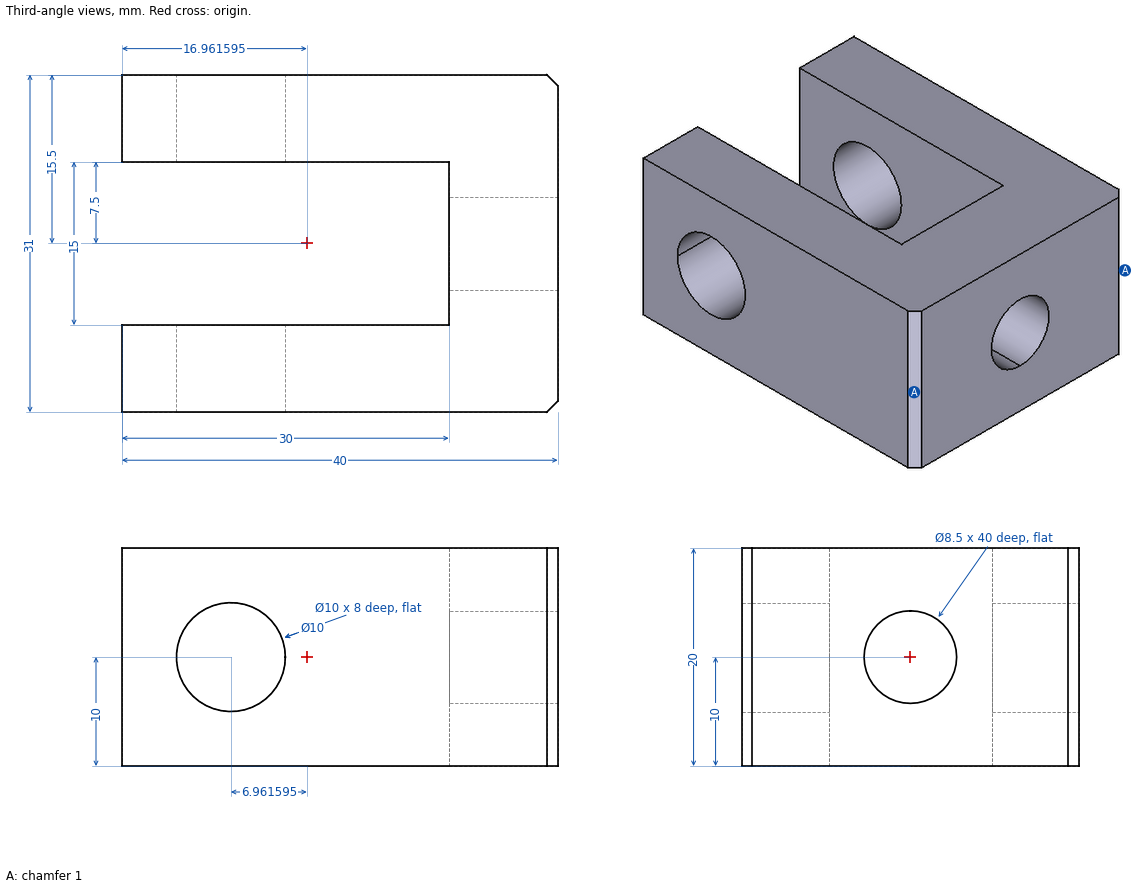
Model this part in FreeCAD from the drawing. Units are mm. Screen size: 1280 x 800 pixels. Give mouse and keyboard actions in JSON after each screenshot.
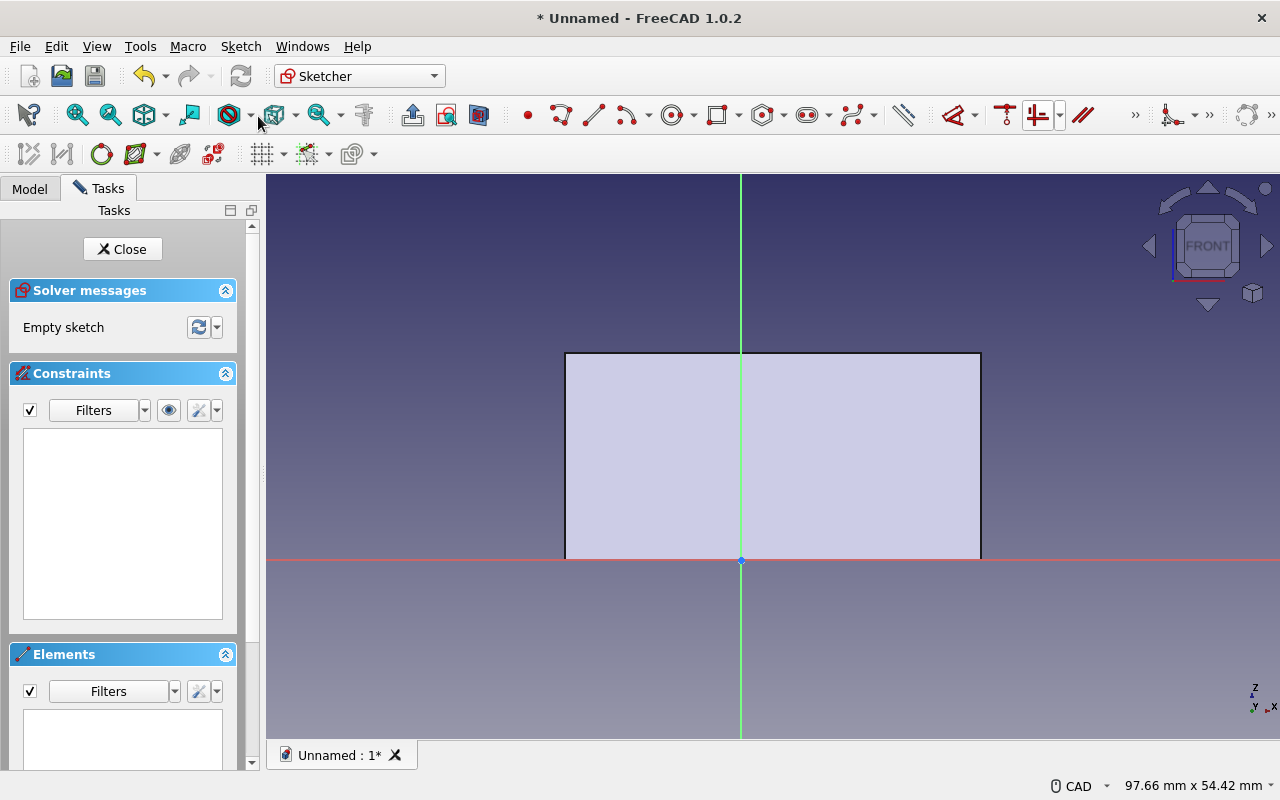
{"action": "scroll", "coordinate": [659, 504], "scroll_direction": "up", "scroll_amount": 4}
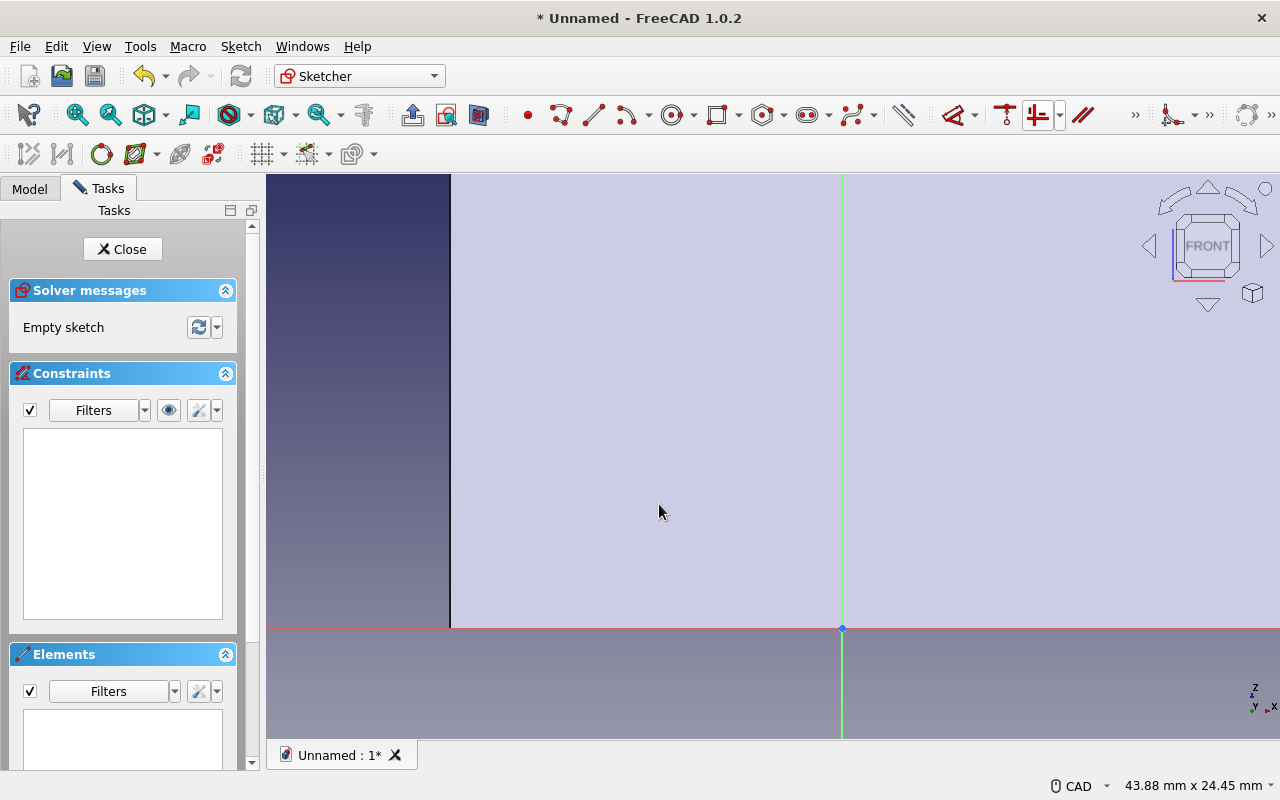
{"action": "key", "text": "g c"}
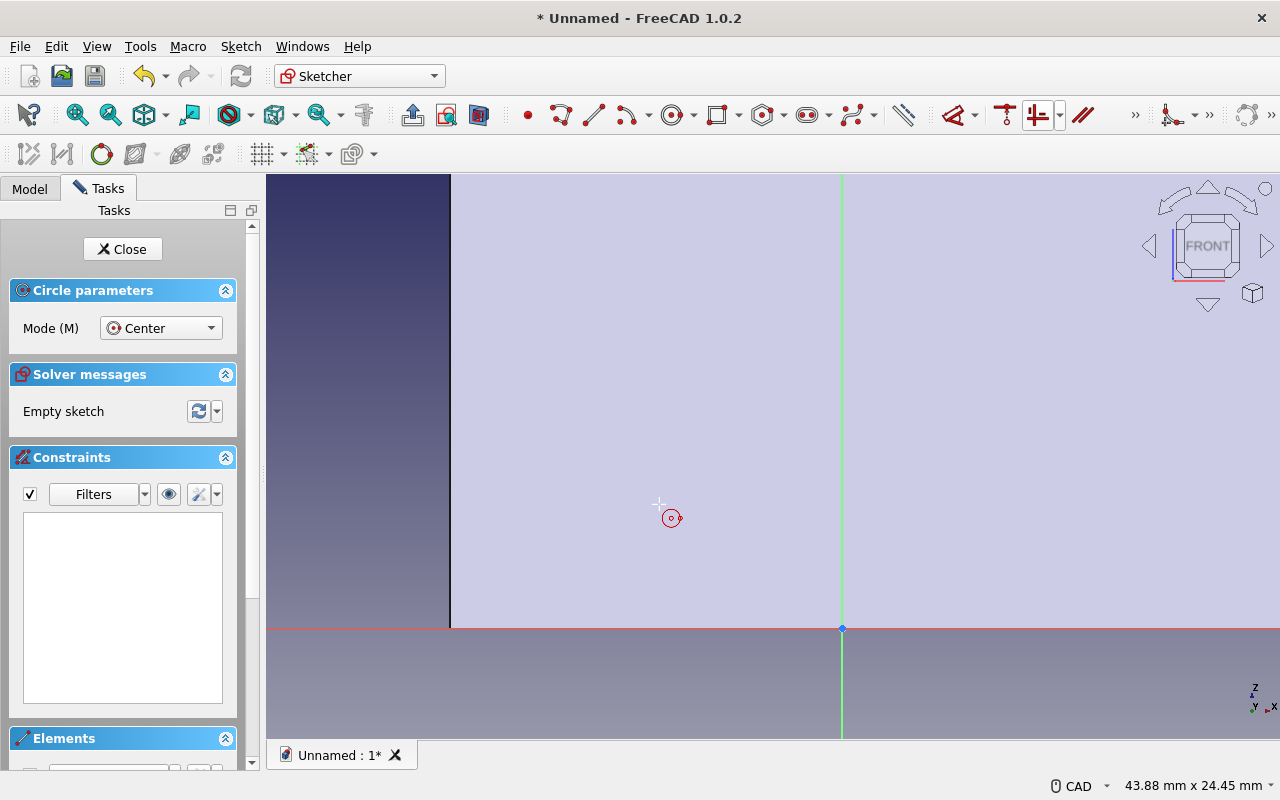
{"action": "left_click", "coordinate": [681, 398]}
{"action": "left_click", "coordinate": [763, 316]}
{"action": "key", "text": "Escape"}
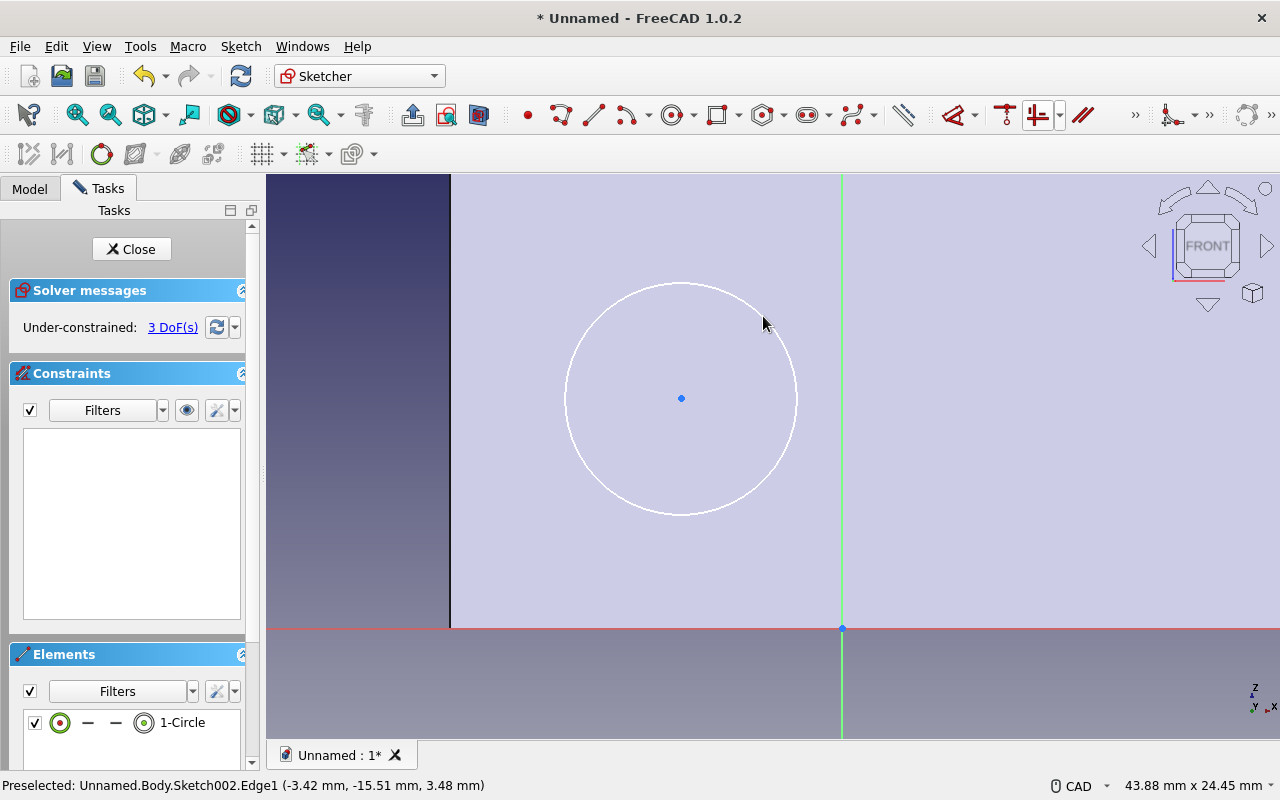
{"action": "key", "text": "d"}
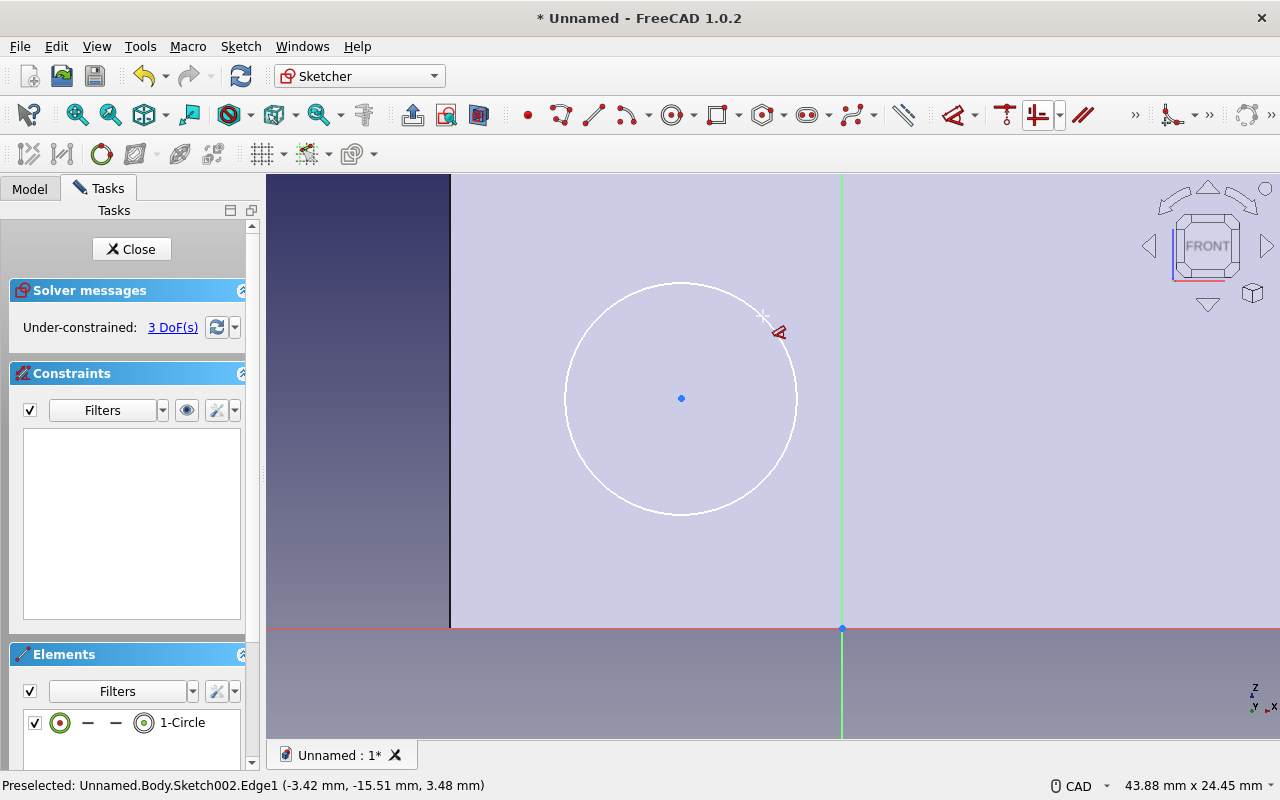
{"action": "left_click", "coordinate": [763, 317]}
{"action": "left_click", "coordinate": [786, 294]}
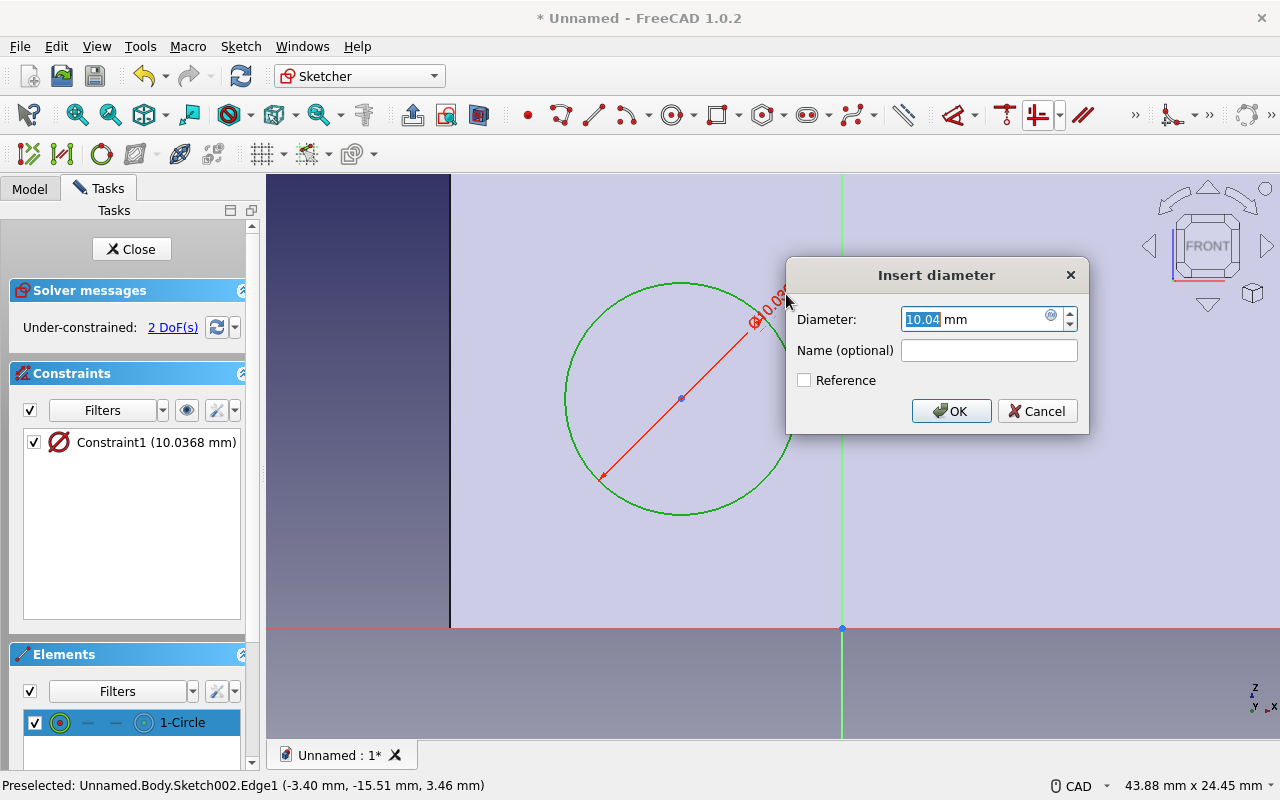
{"action": "type", "text": "10"}
{"action": "key", "text": "Return"}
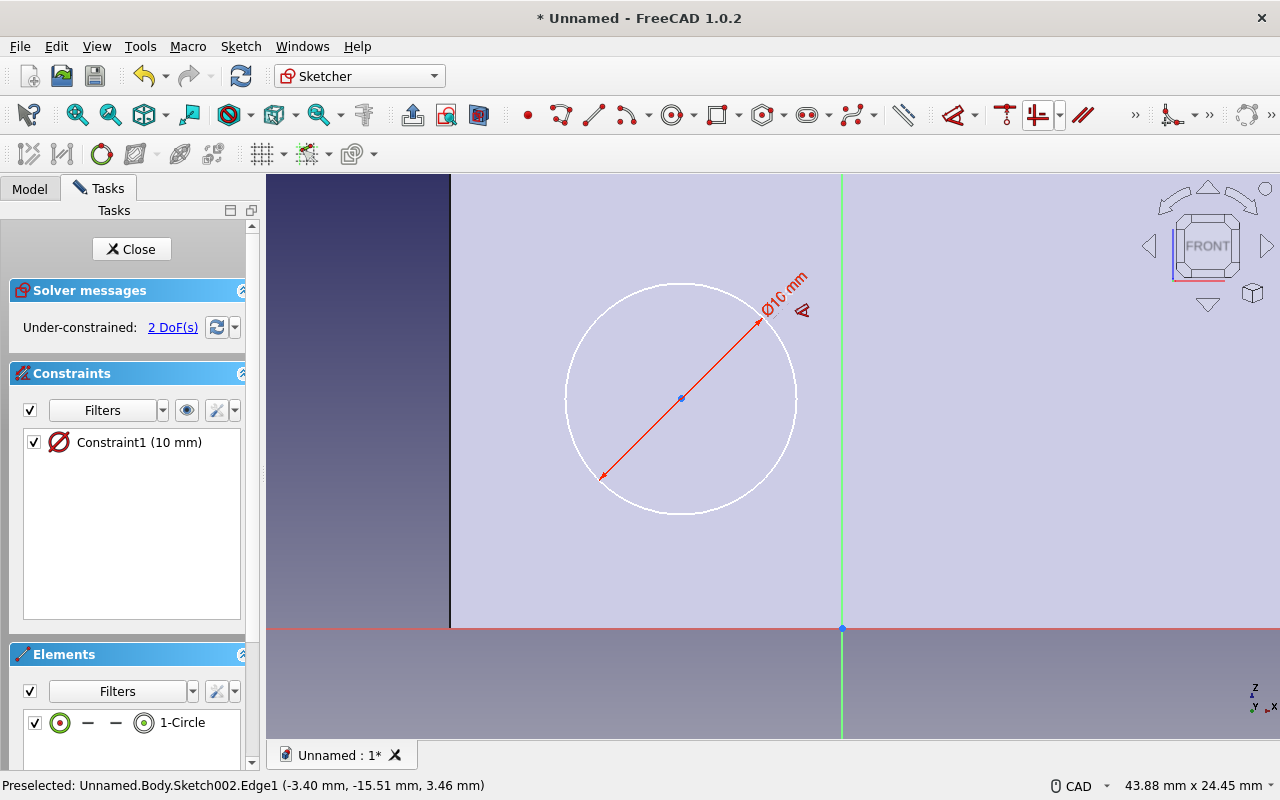
{"action": "left_click", "coordinate": [681, 399]}
{"action": "left_click", "coordinate": [876, 514]}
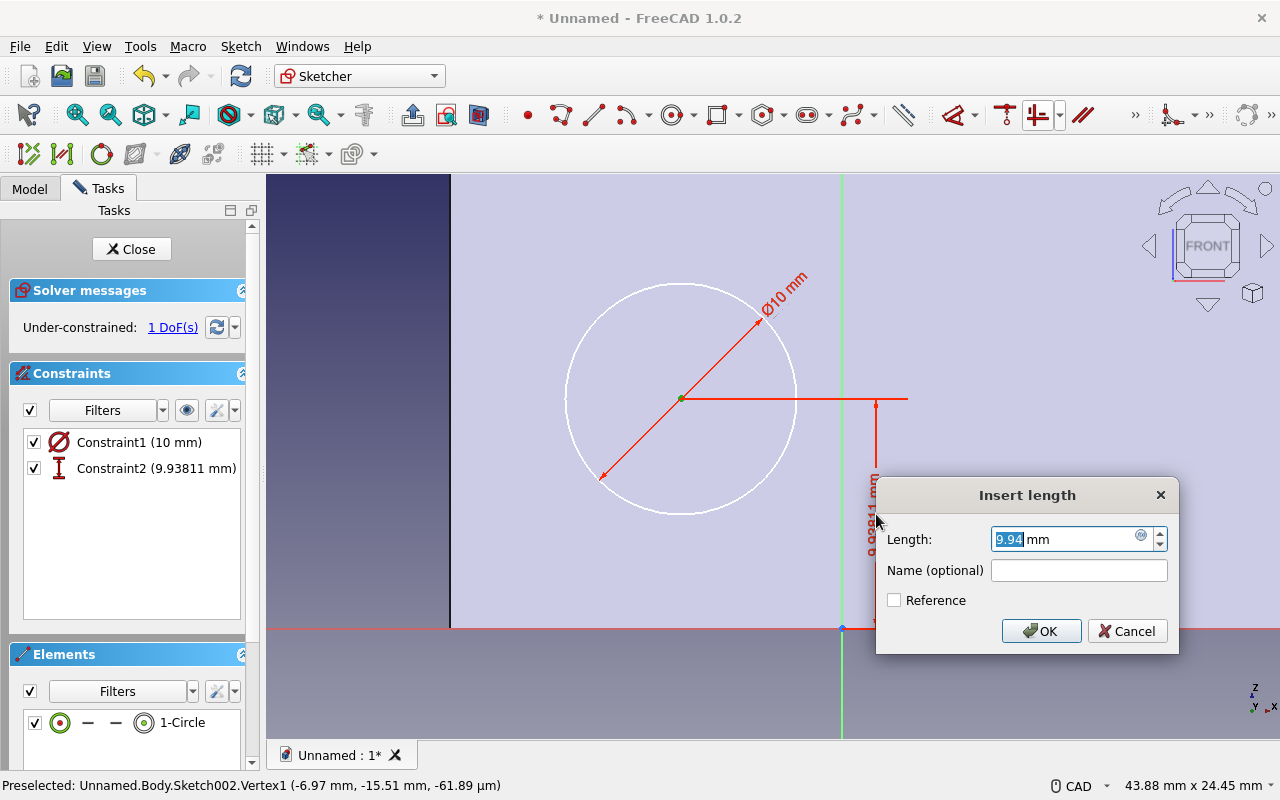
{"action": "type", "text": "10"}
{"action": "key", "text": "Return"}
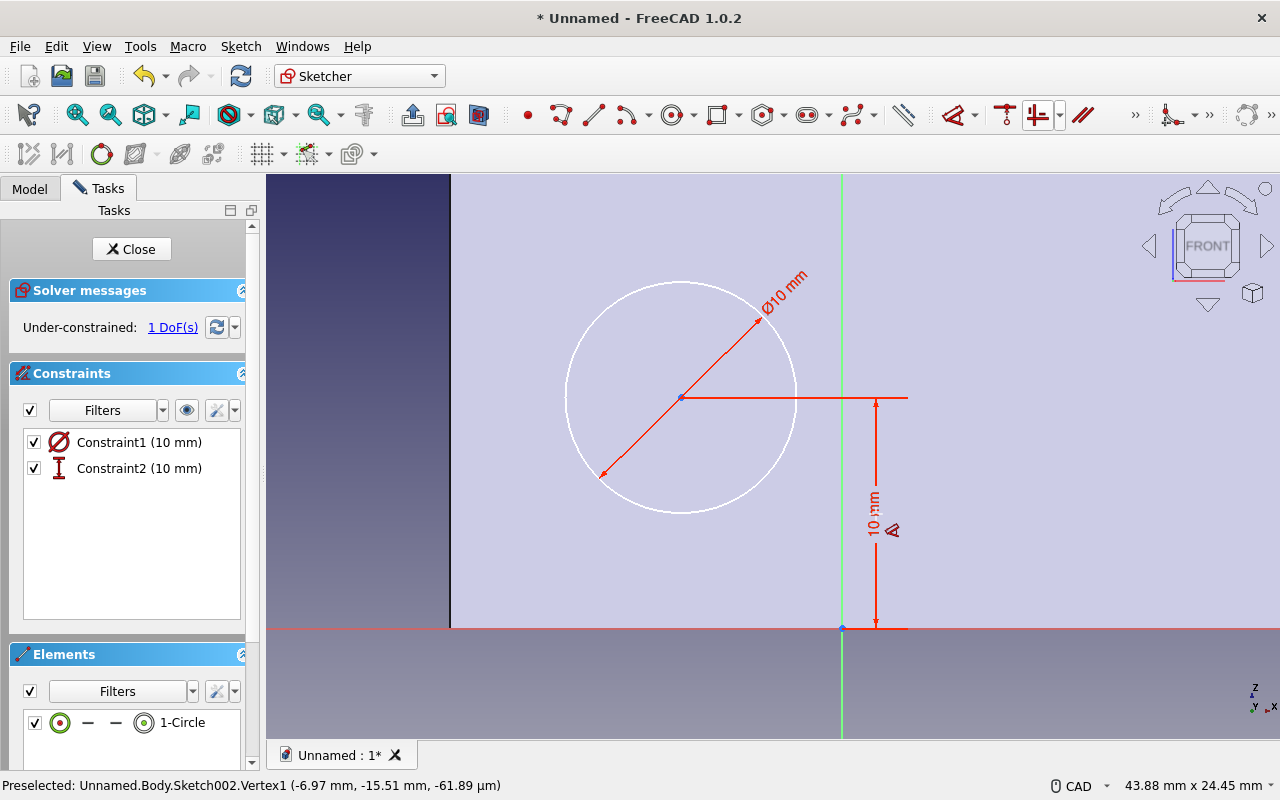
{"action": "left_click", "coordinate": [681, 398]}
{"action": "left_click", "coordinate": [762, 663]}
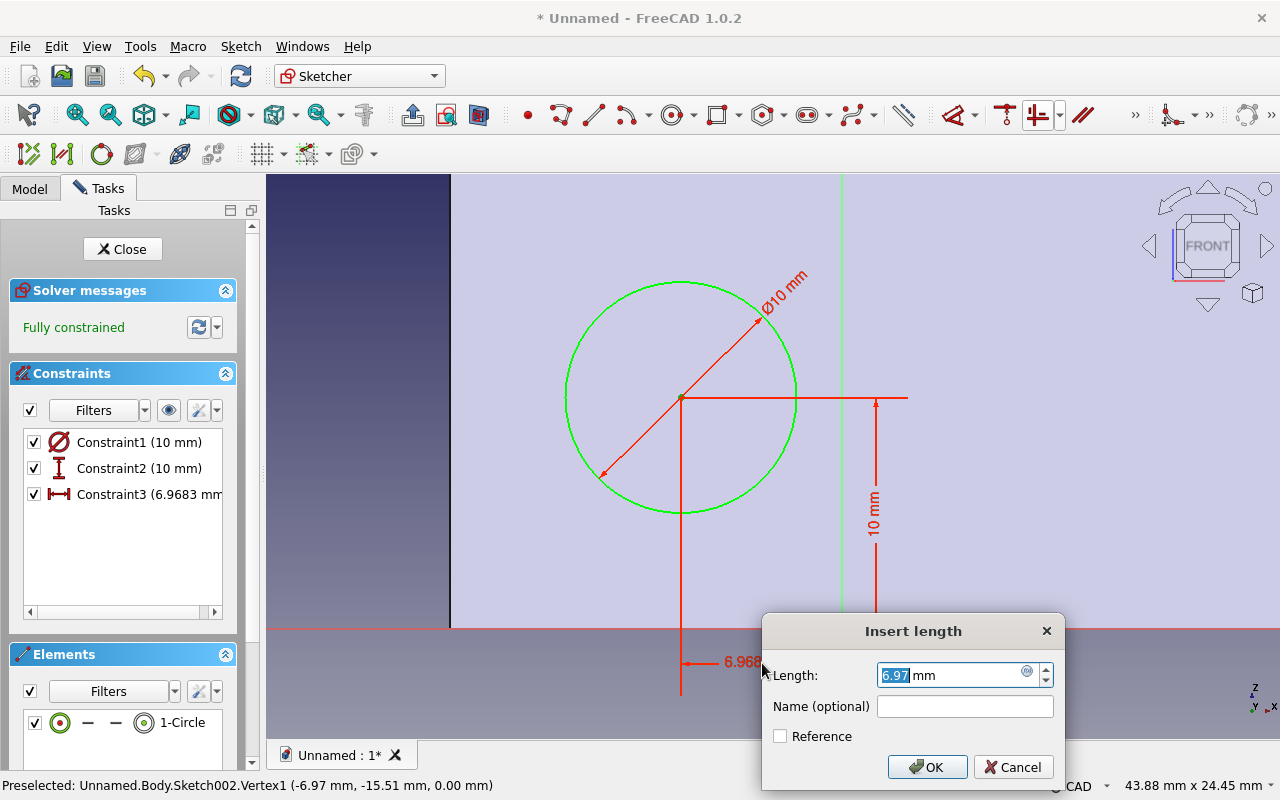
{"action": "type", "text": "6.961595"}
{"action": "key", "text": "Return"}
{"action": "key", "text": "Escape"}